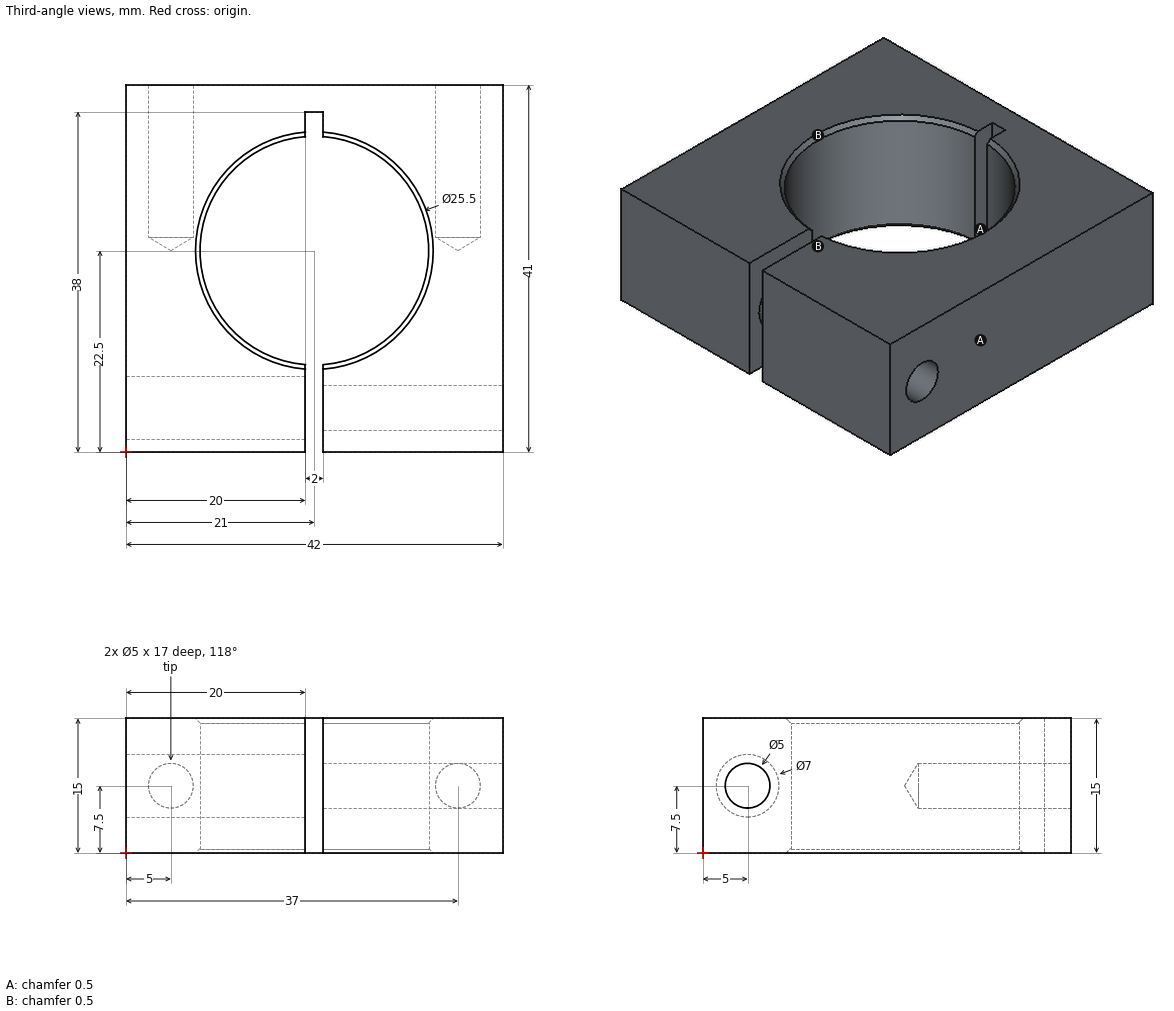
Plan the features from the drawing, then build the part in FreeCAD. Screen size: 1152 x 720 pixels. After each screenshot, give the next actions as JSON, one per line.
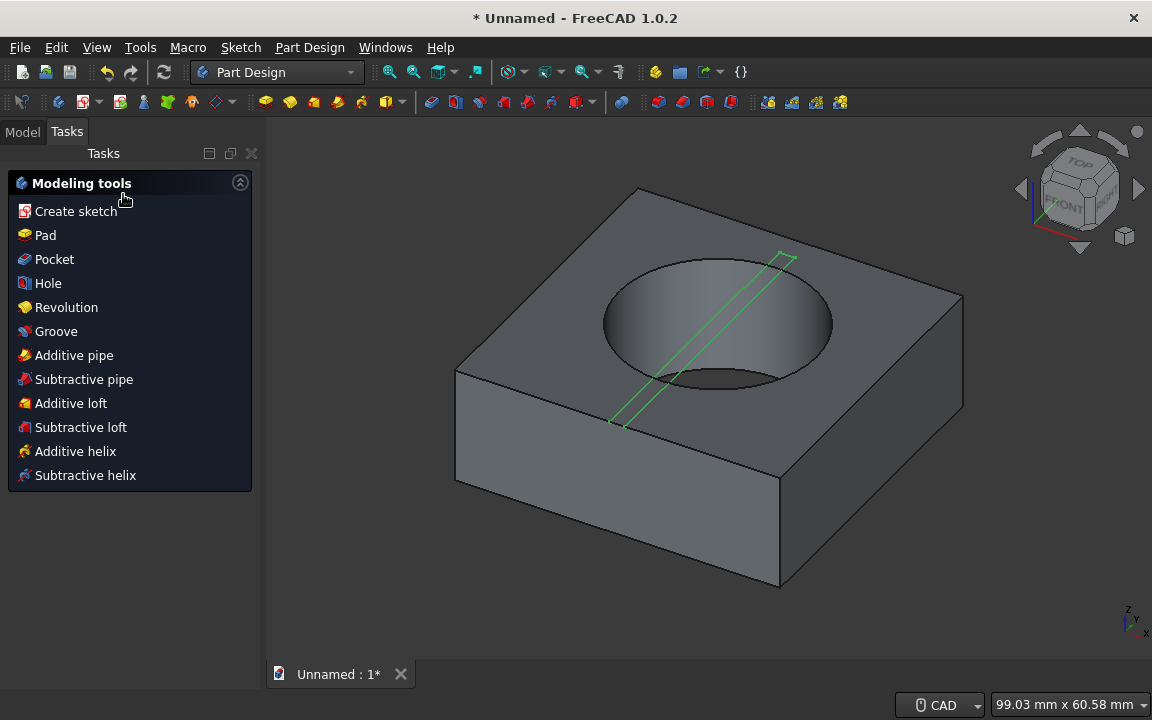
{"action": "left_click", "coordinate": [432, 102]}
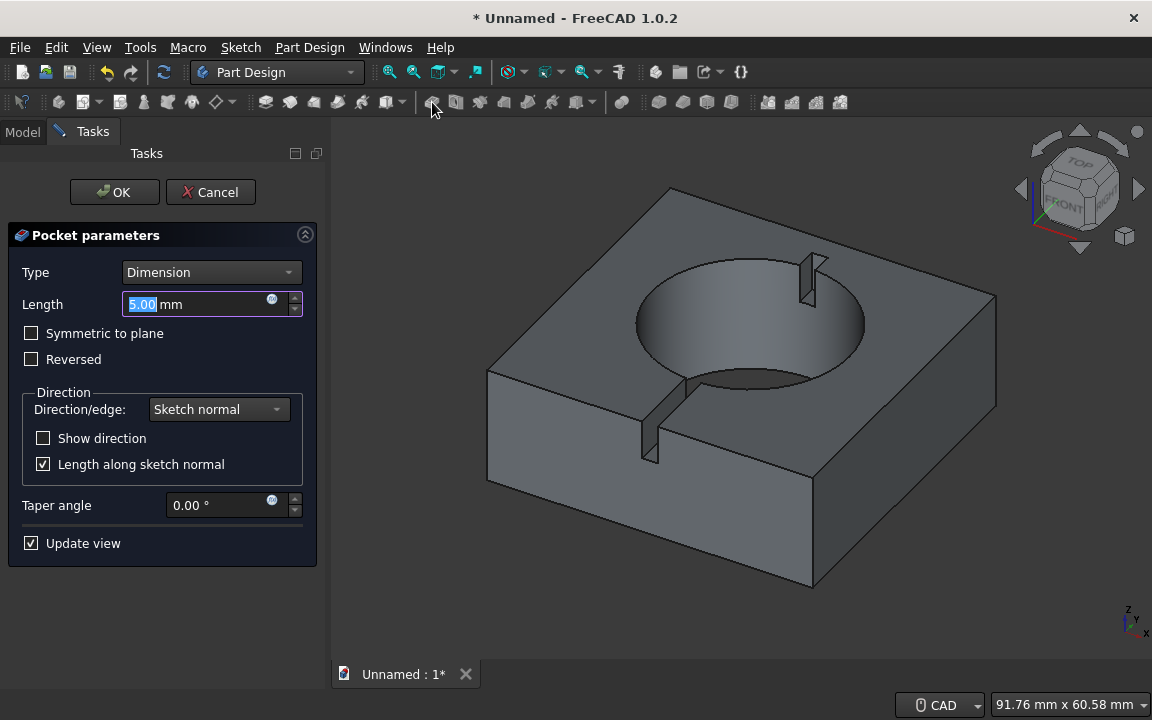
{"action": "type", "text": "15"}
{"action": "key", "text": "Tab"}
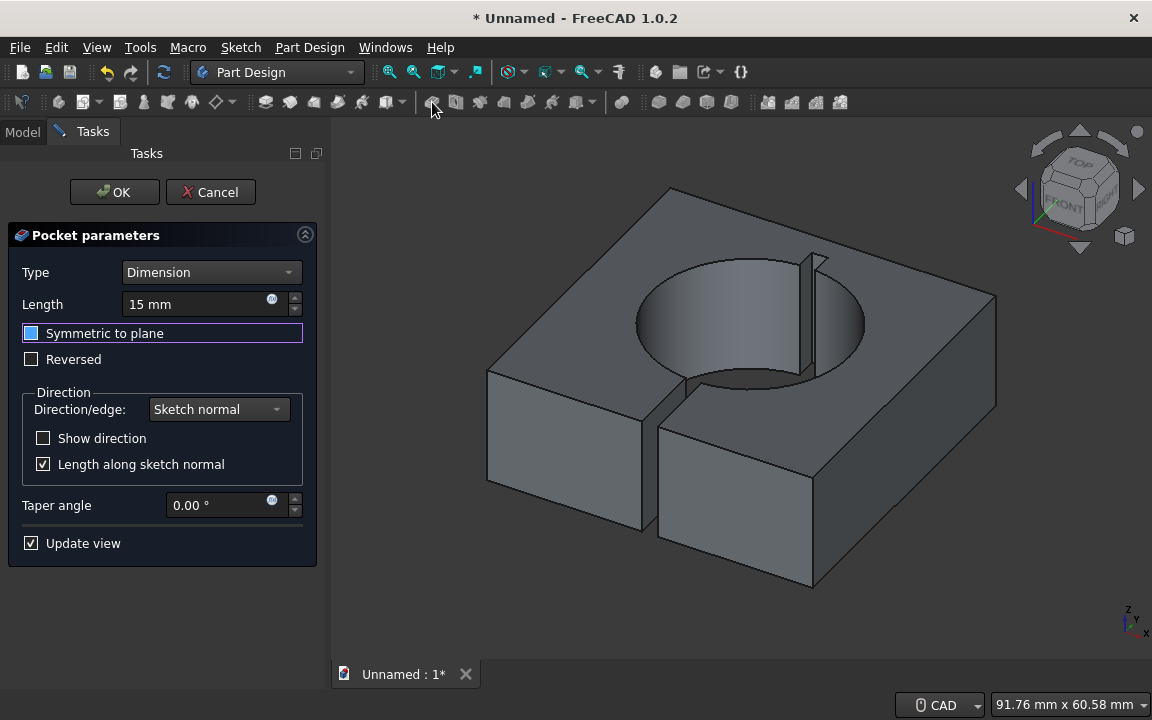
{"action": "left_click", "coordinate": [115, 192]}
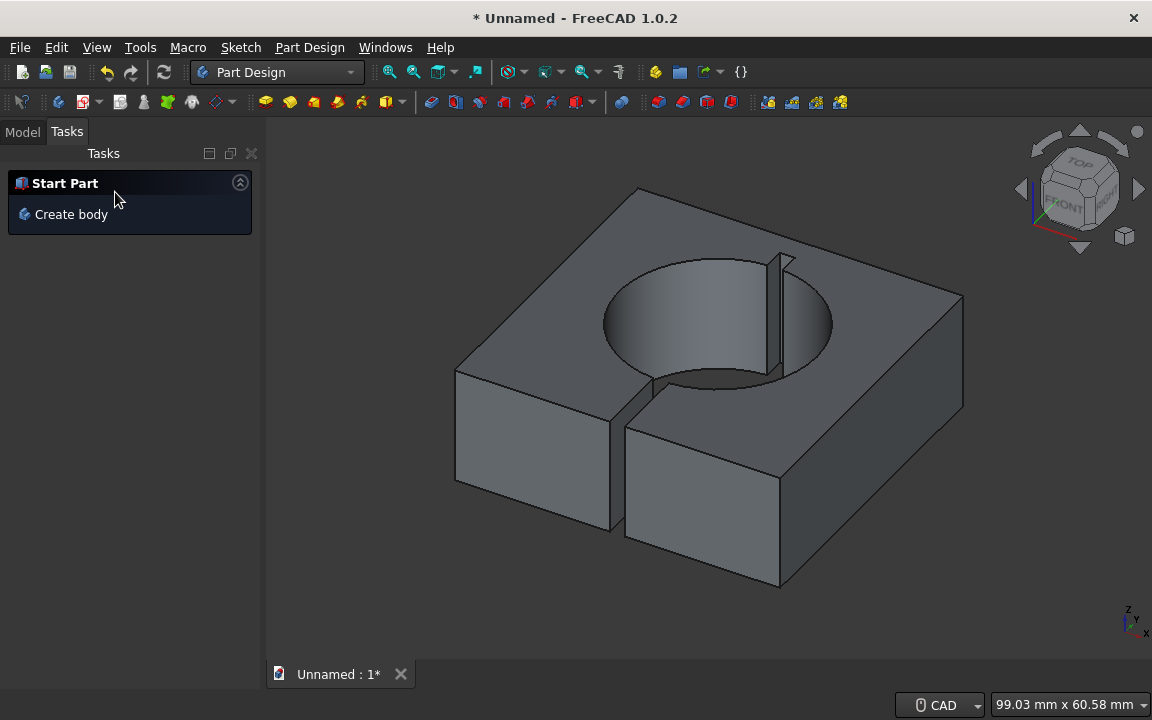
{"action": "key", "text": "4"}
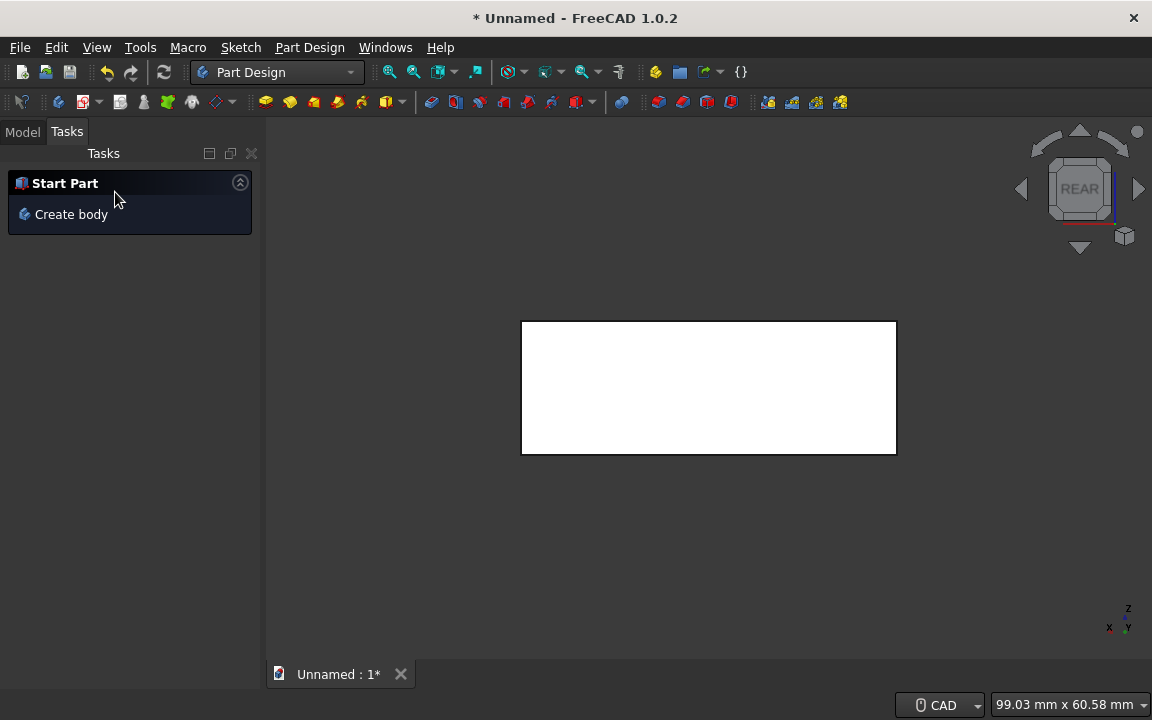
{"action": "left_click", "coordinate": [390, 72]}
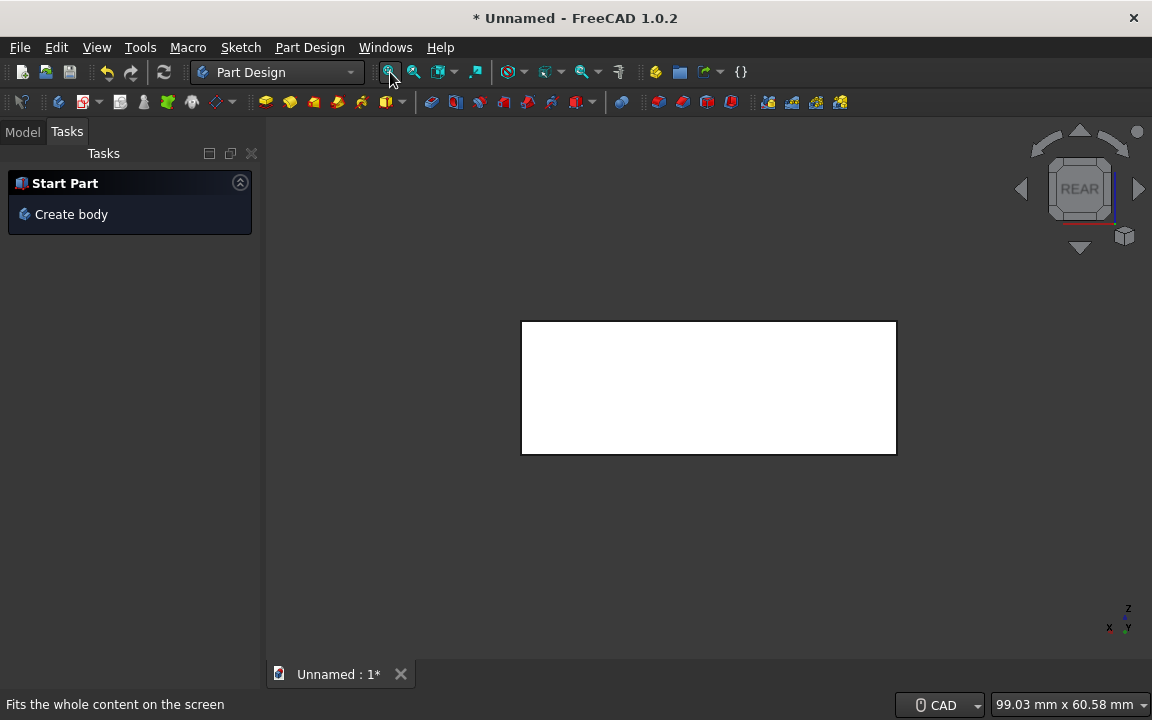
{"action": "left_click", "coordinate": [602, 387]}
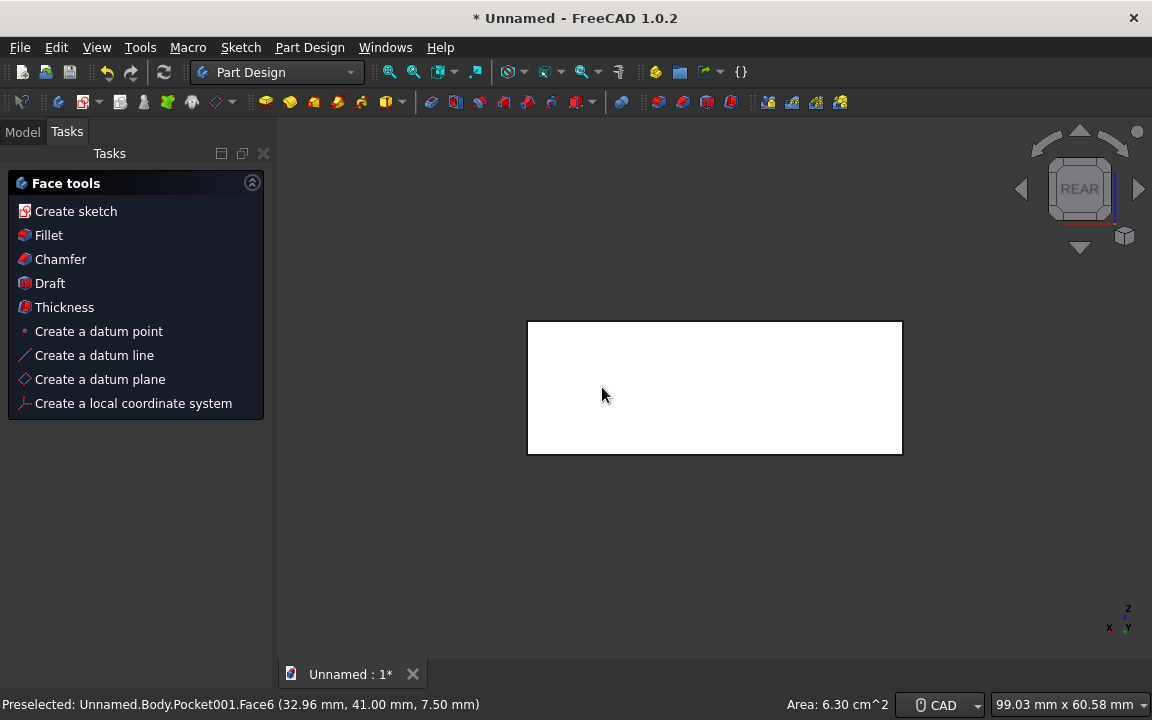
{"action": "left_click", "coordinate": [84, 102]}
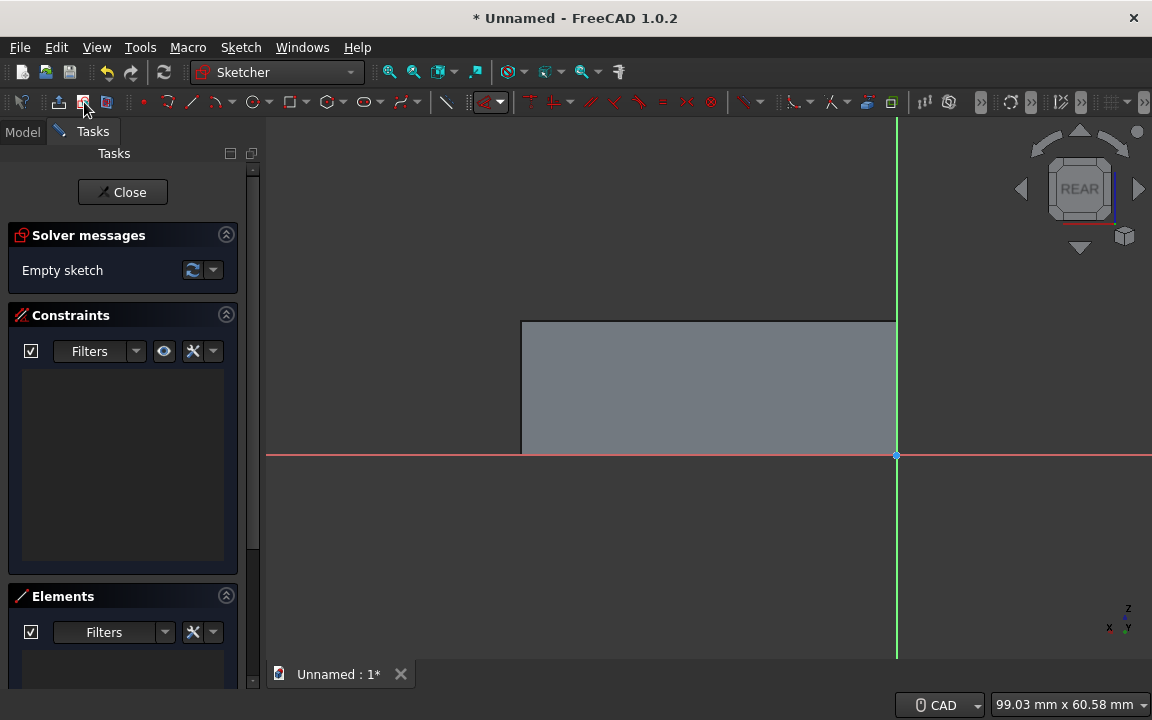
{"action": "scroll", "coordinate": [882, 456], "scroll_direction": "up", "scroll_amount": 2}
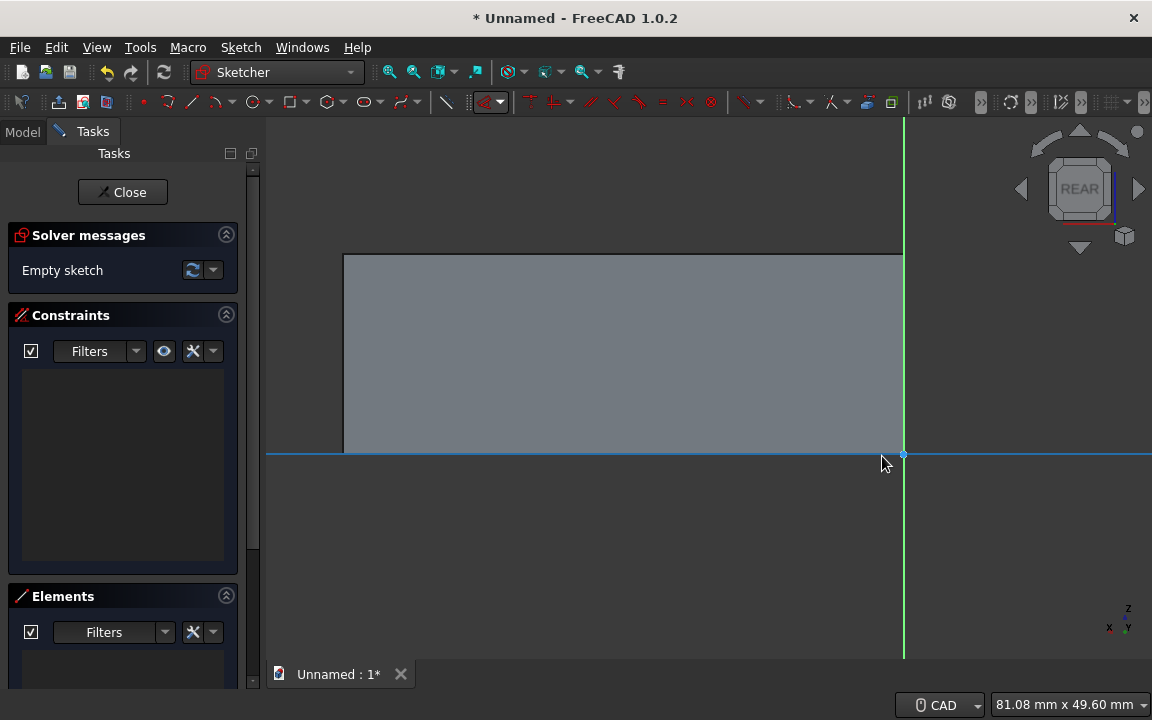
{"action": "left_click", "coordinate": [254, 102]}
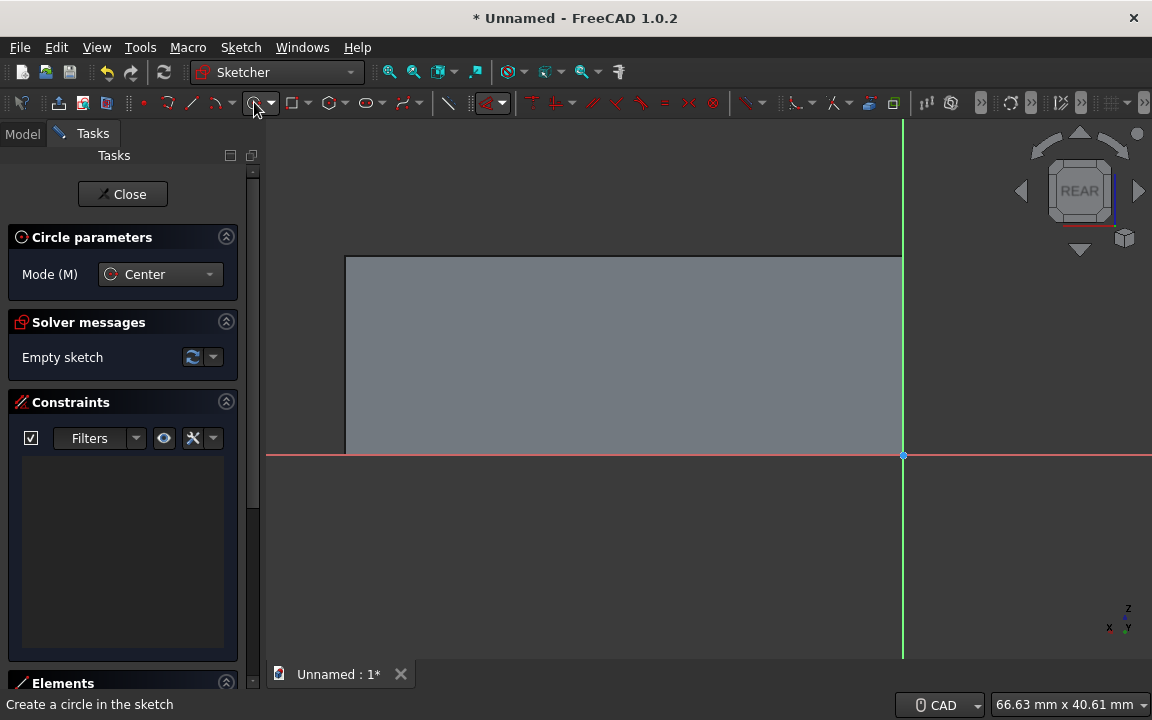
{"action": "left_click", "coordinate": [837, 355]}
{"action": "mouse_move", "coordinate": [860, 332]}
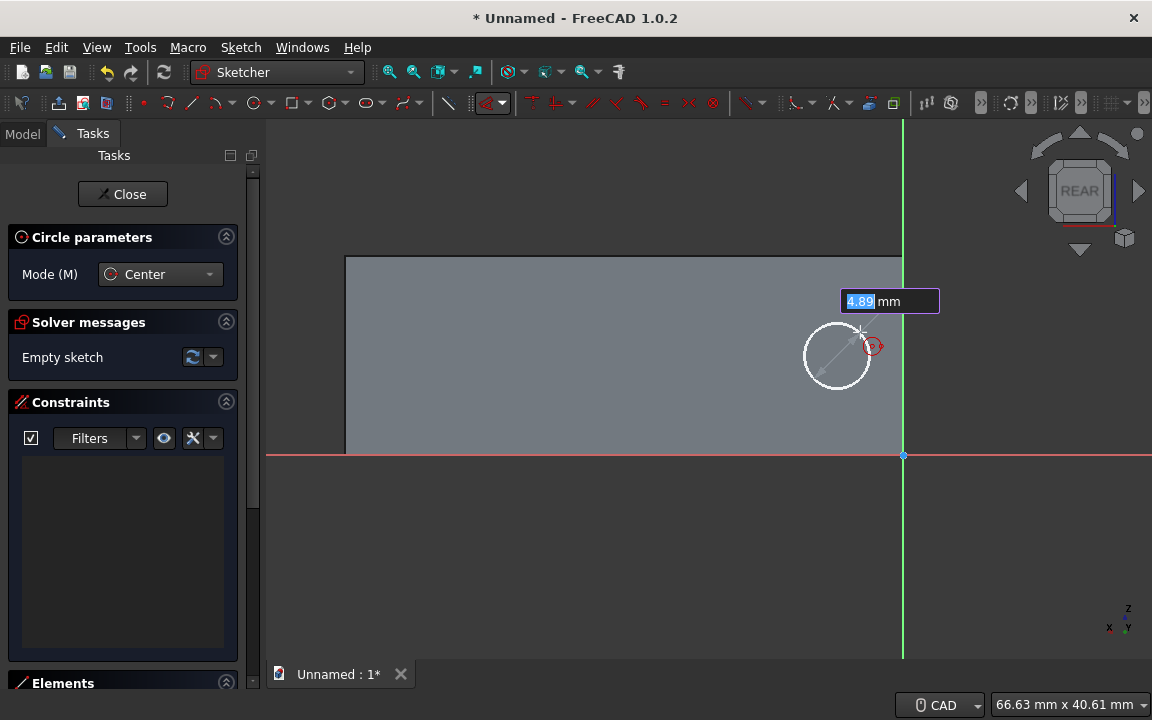
{"action": "type", "text": "5"}
{"action": "key", "text": "Return"}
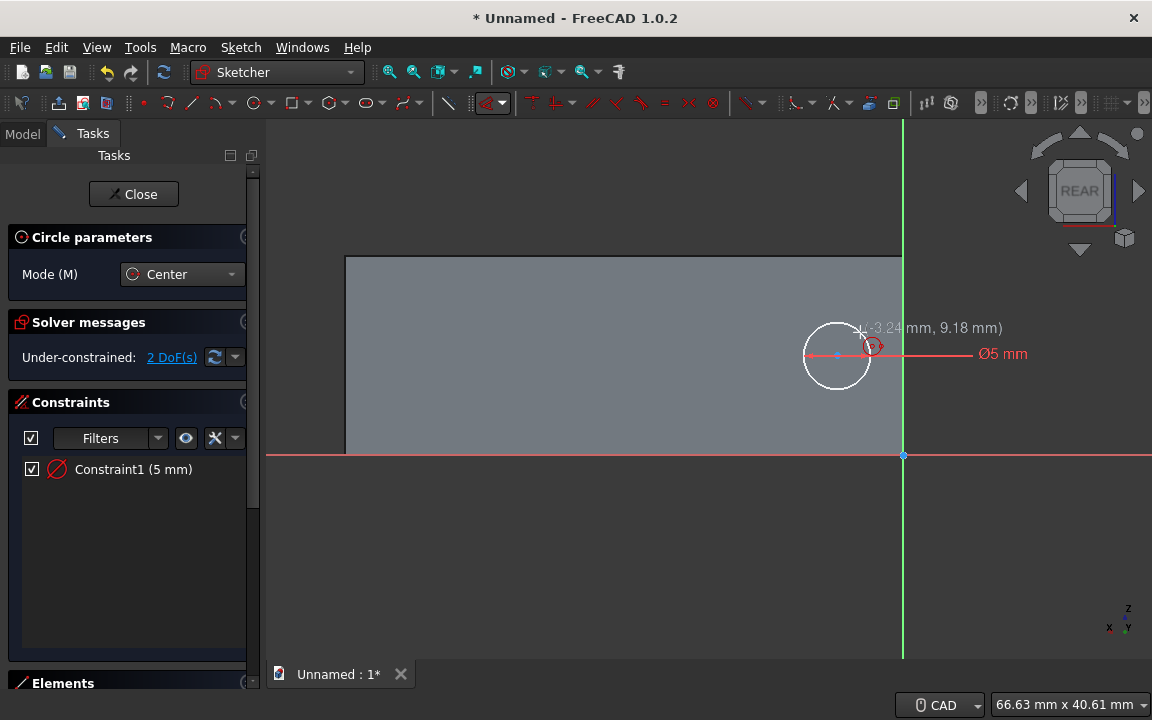
{"action": "left_click", "coordinate": [411, 355]}
{"action": "mouse_move", "coordinate": [435, 332]}